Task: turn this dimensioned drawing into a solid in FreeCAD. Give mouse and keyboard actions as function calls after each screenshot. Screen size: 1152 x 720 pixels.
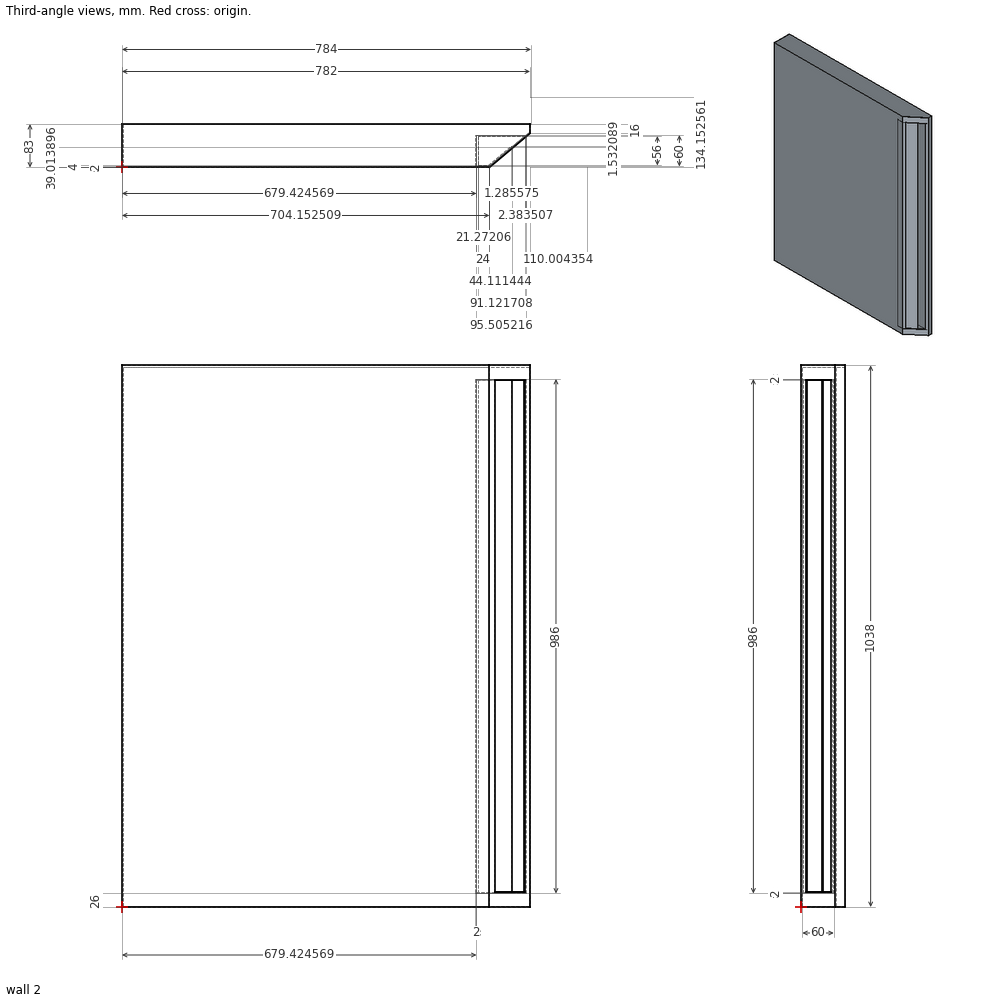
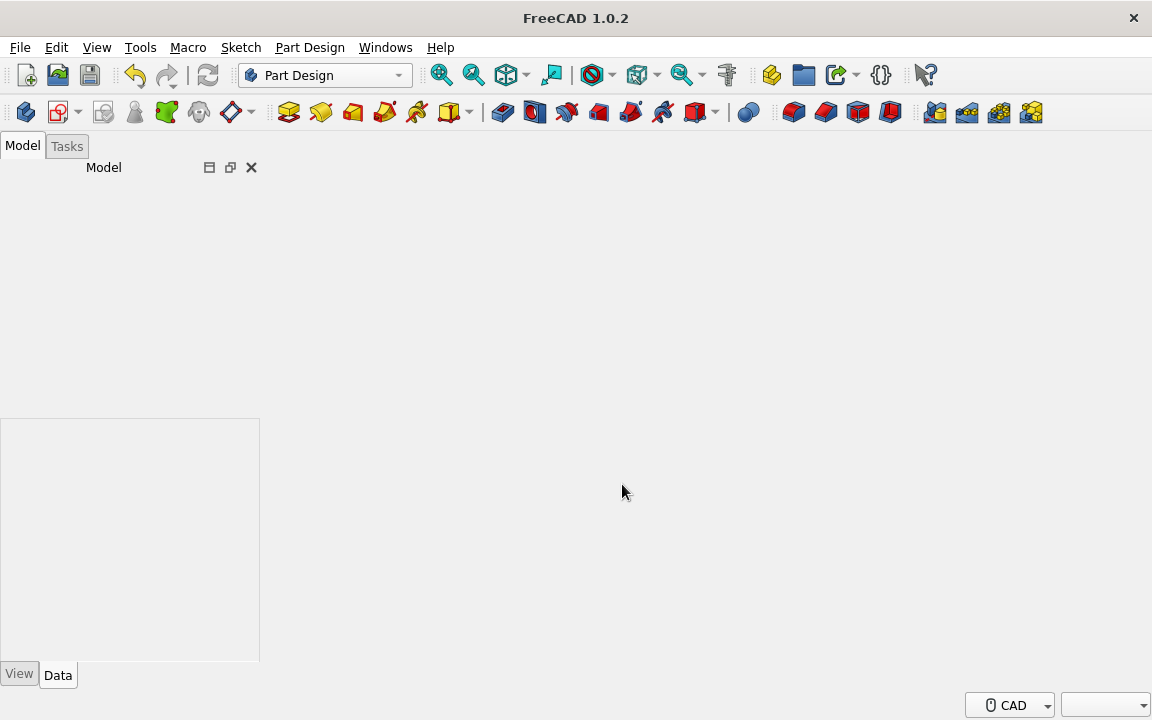
click(26, 76)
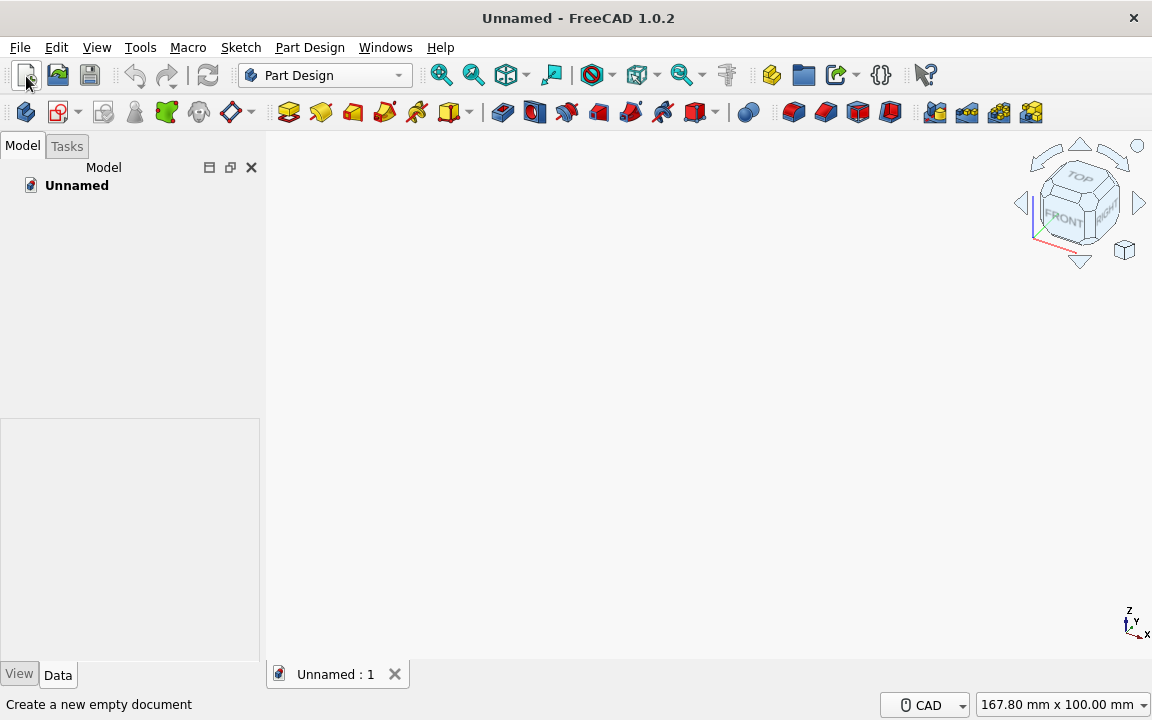
click(58, 112)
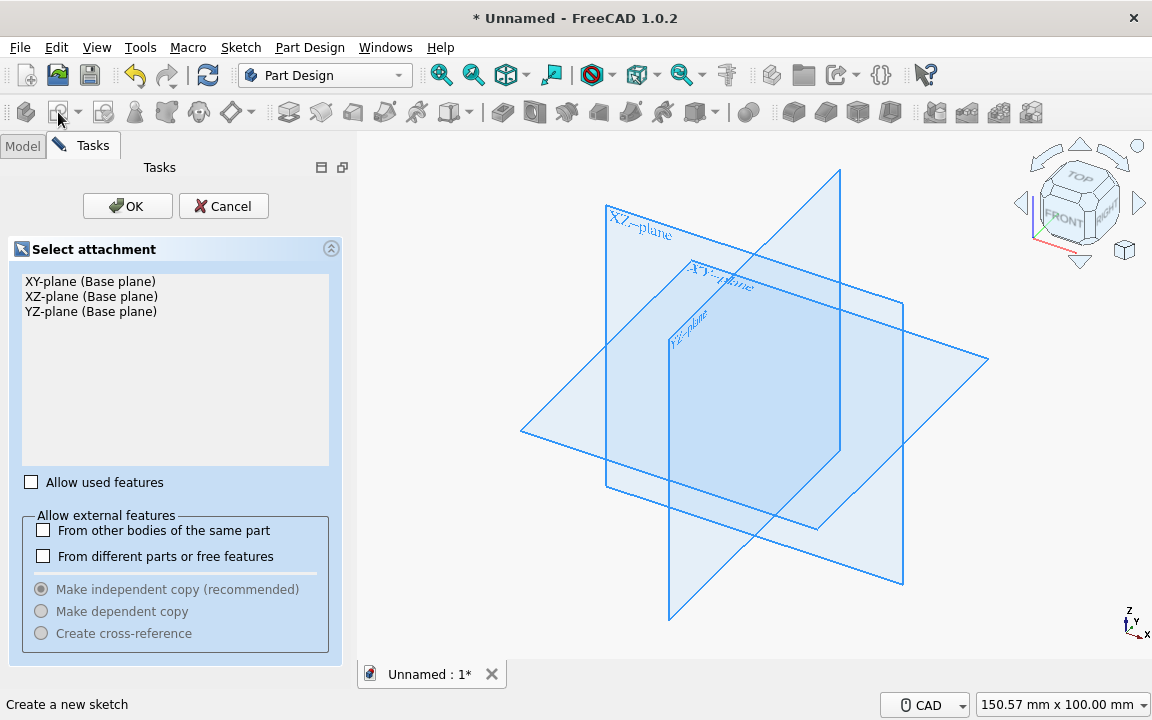
click(82, 282)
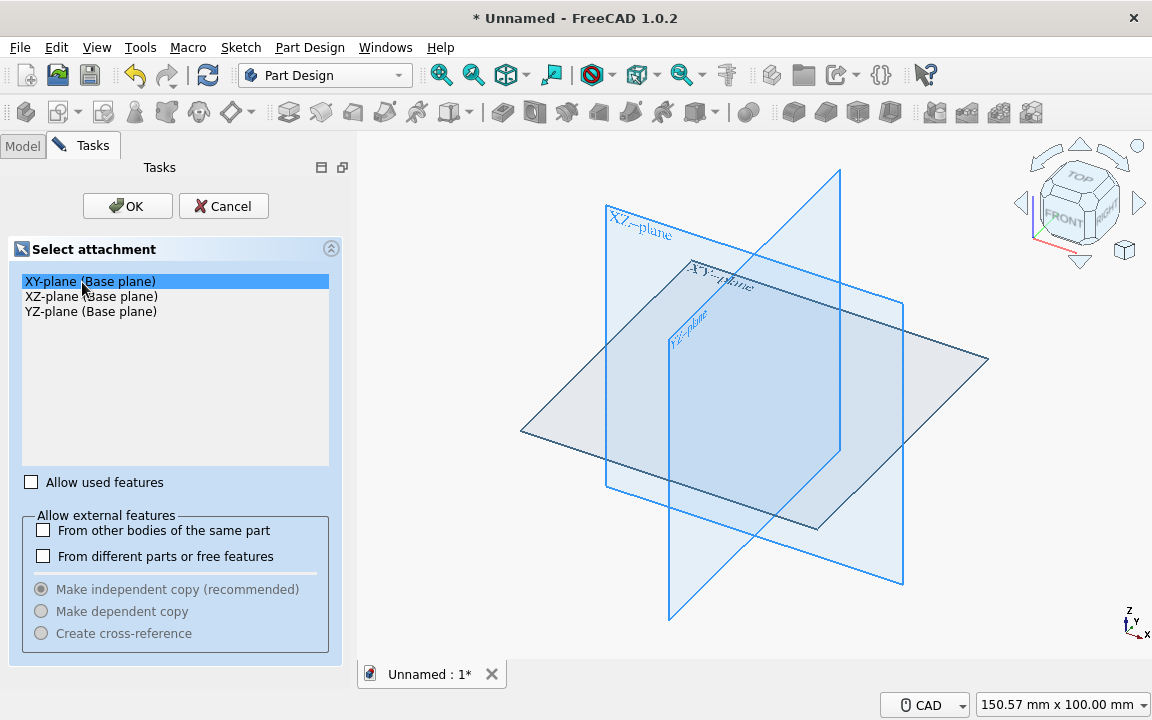
click(128, 206)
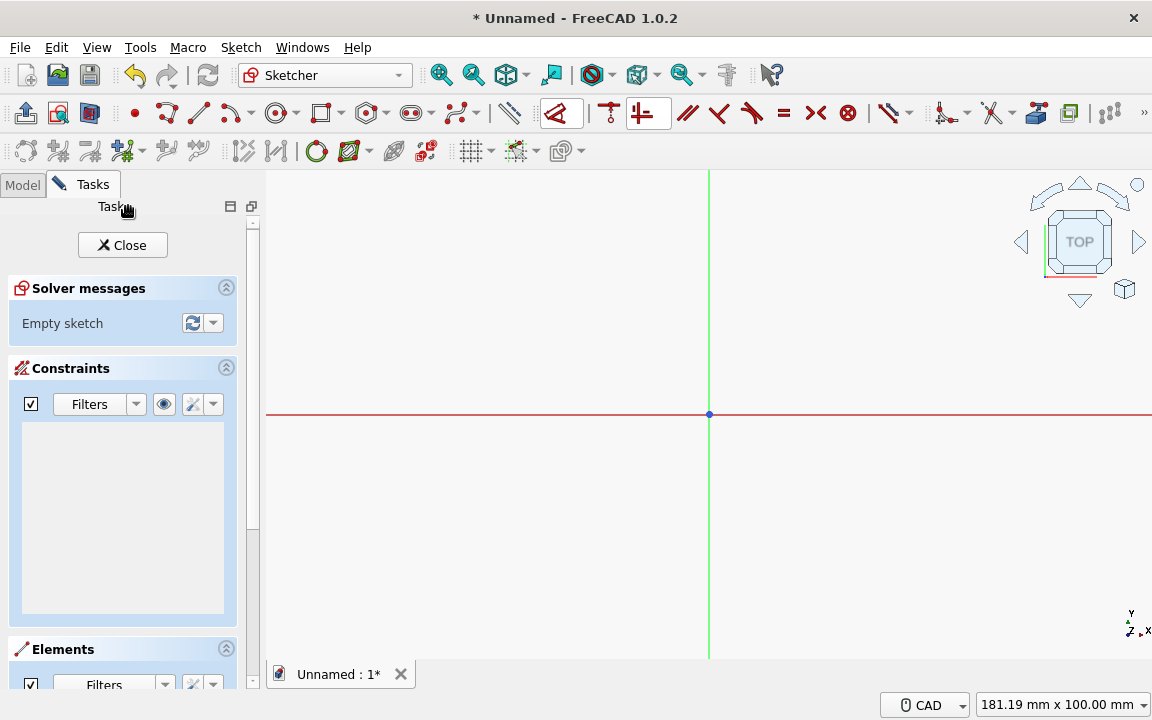
scroll(330, 446, down, 10)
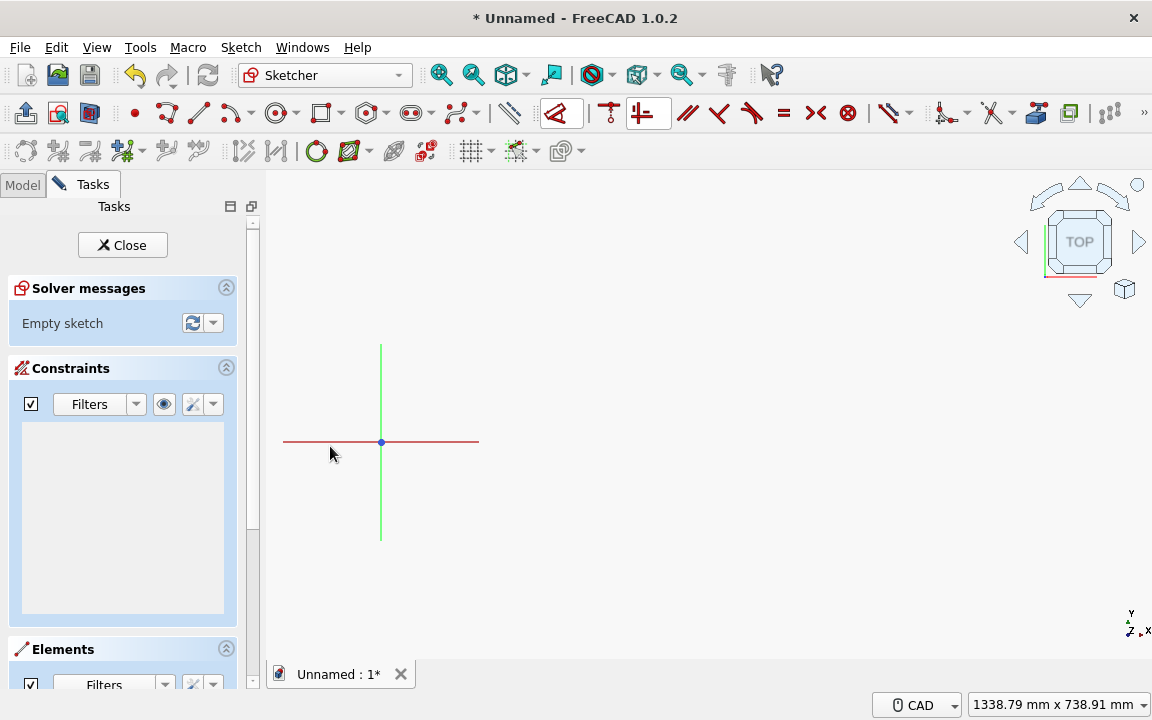
key(g)
key(m)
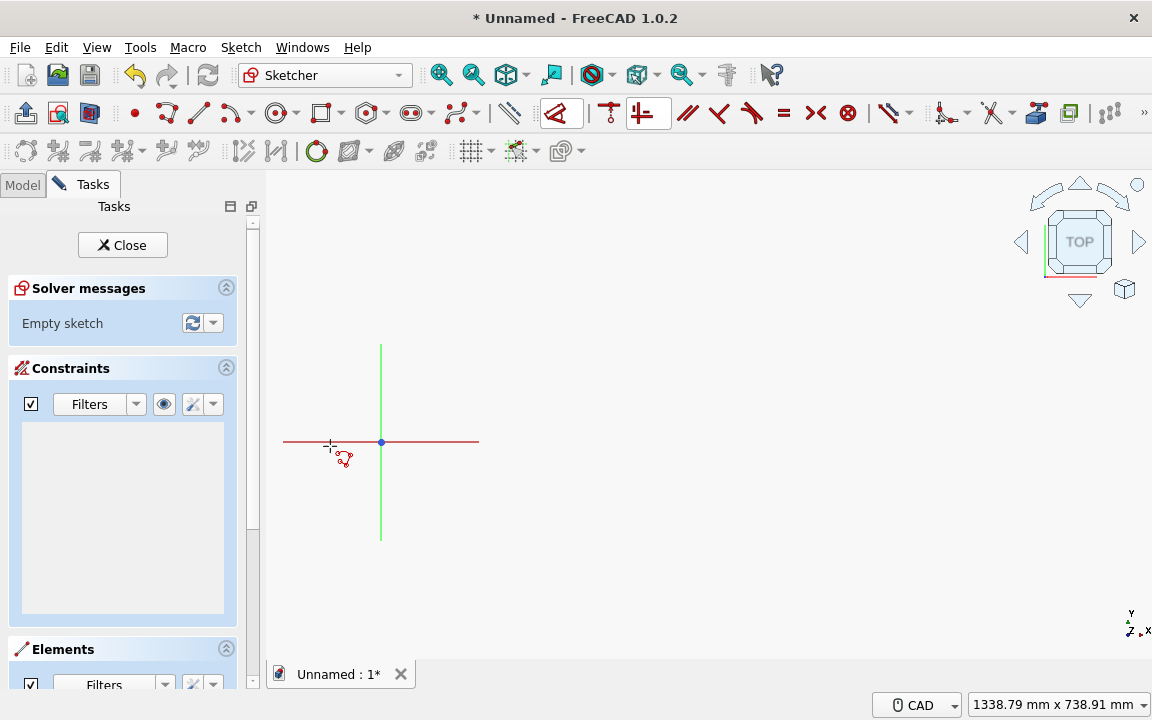
click(381, 442)
click(847, 433)
click(900, 398)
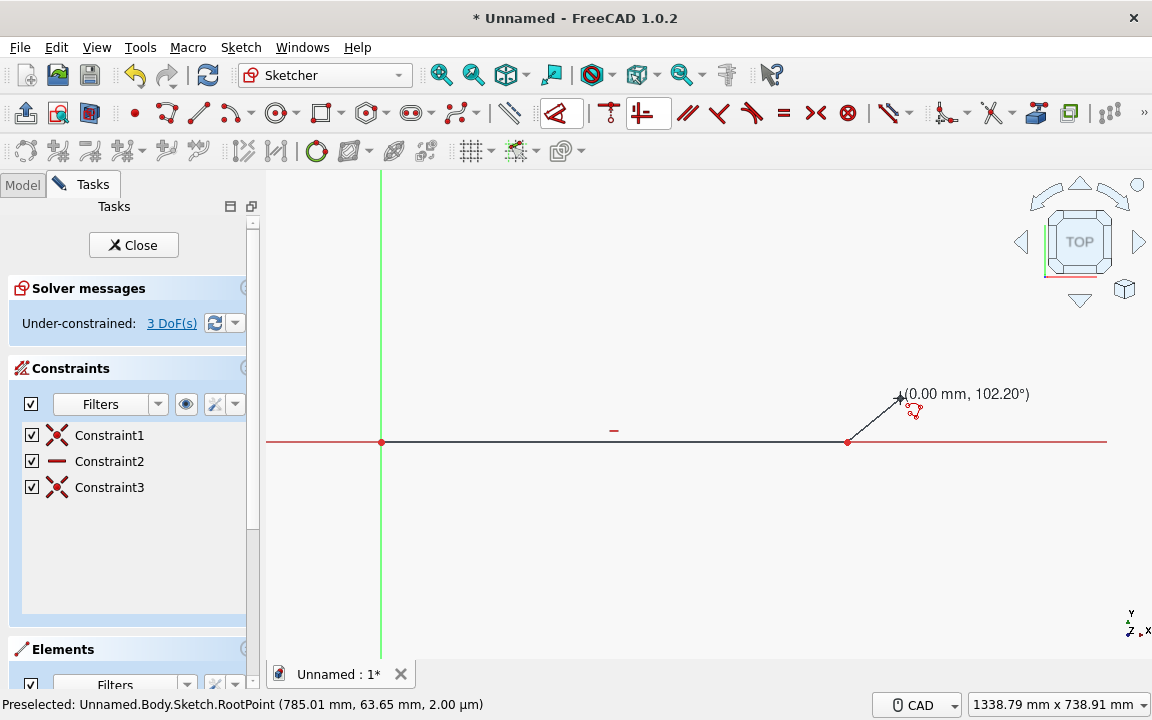
scroll(900, 387, up, 3)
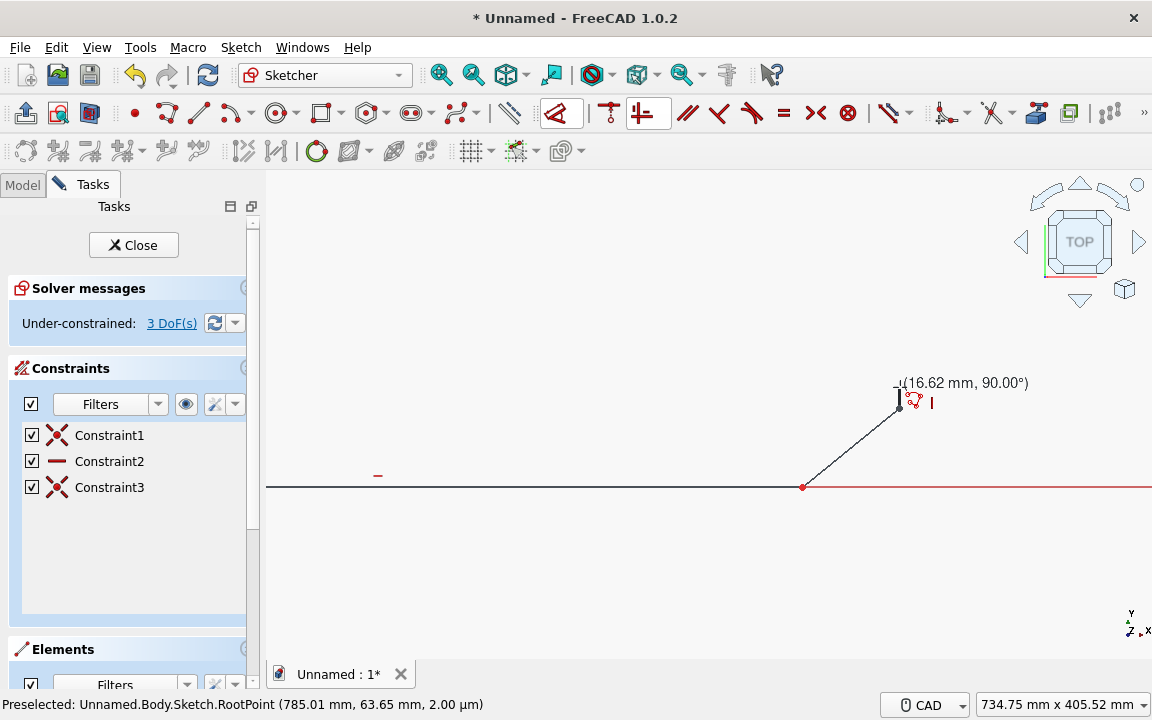
click(899, 387)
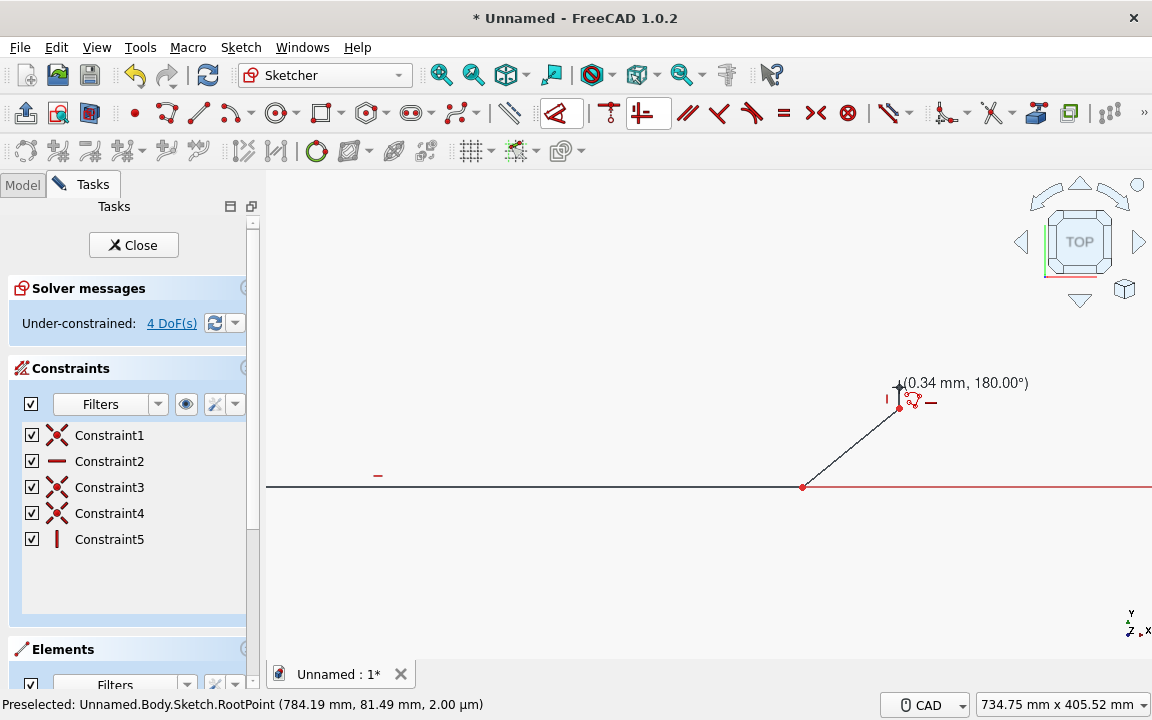
scroll(900, 387, down, 3)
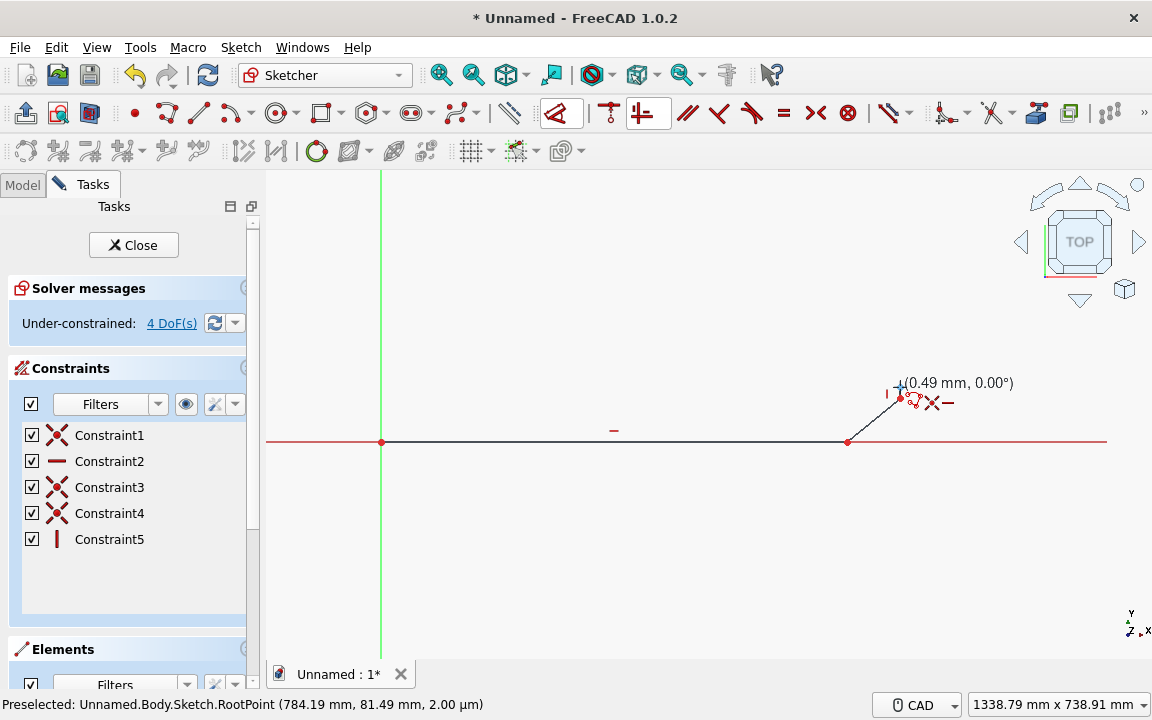
click(390, 387)
click(381, 442)
key(Escape)
key(Escape)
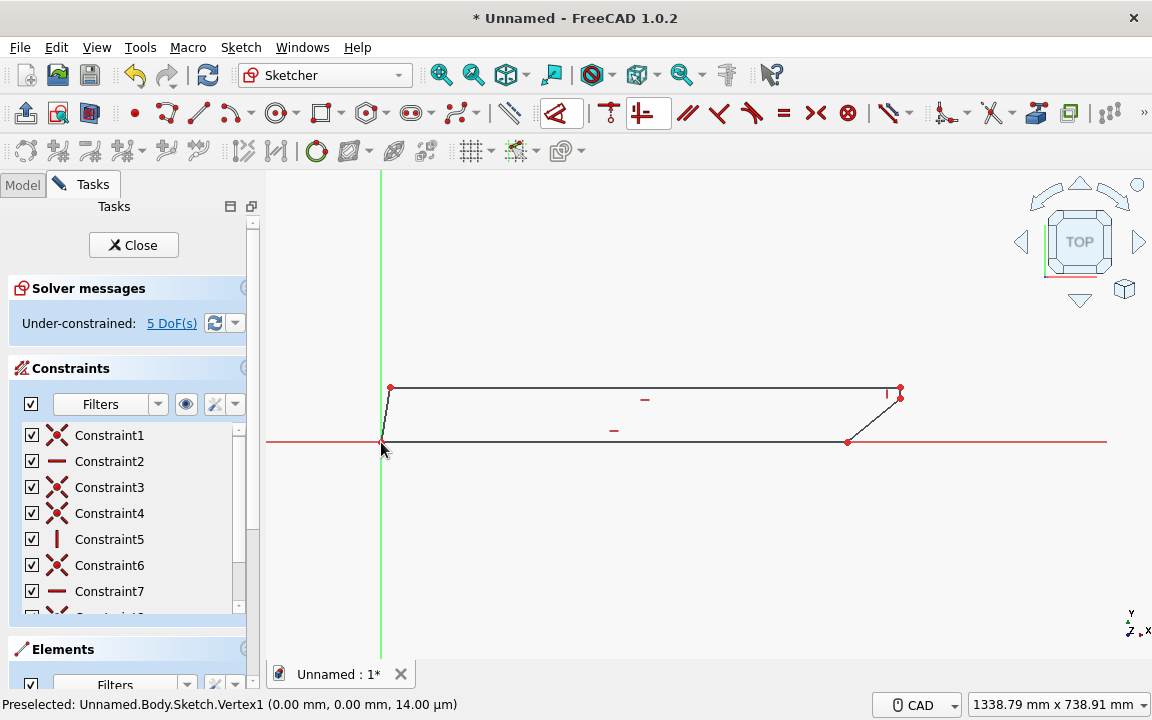
click(384, 426)